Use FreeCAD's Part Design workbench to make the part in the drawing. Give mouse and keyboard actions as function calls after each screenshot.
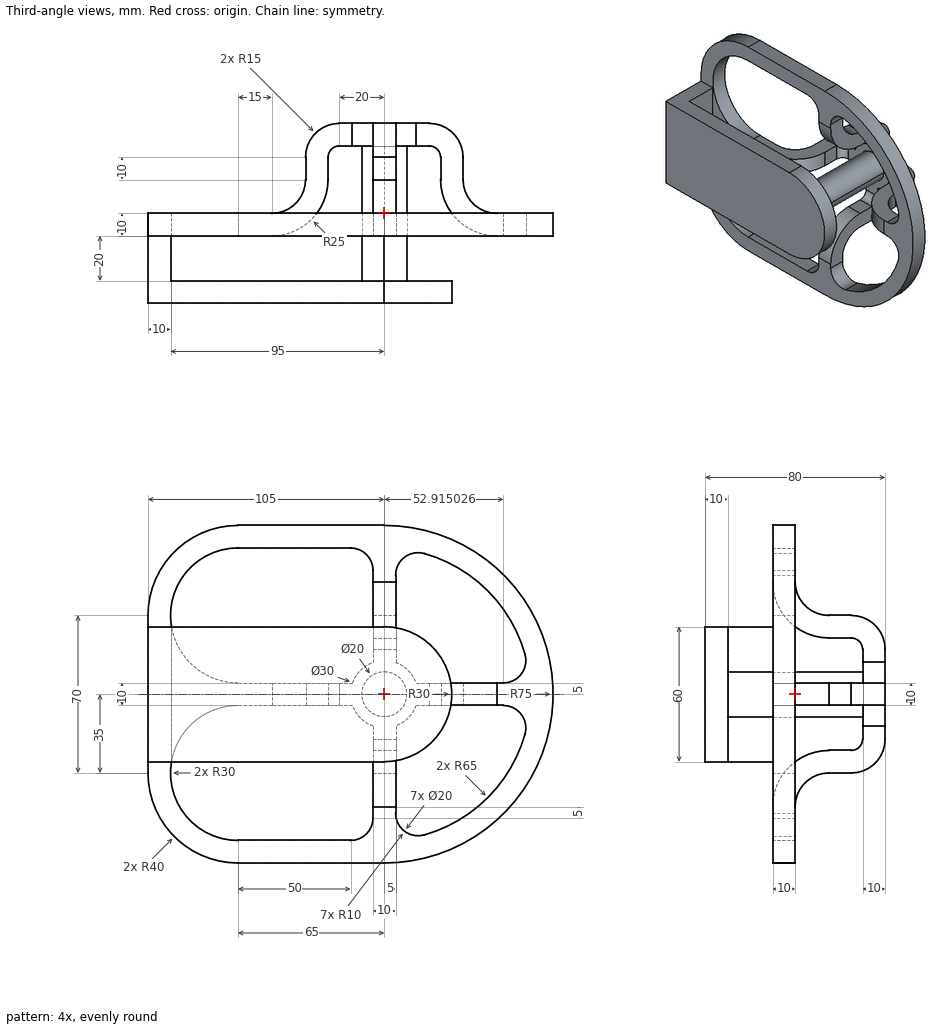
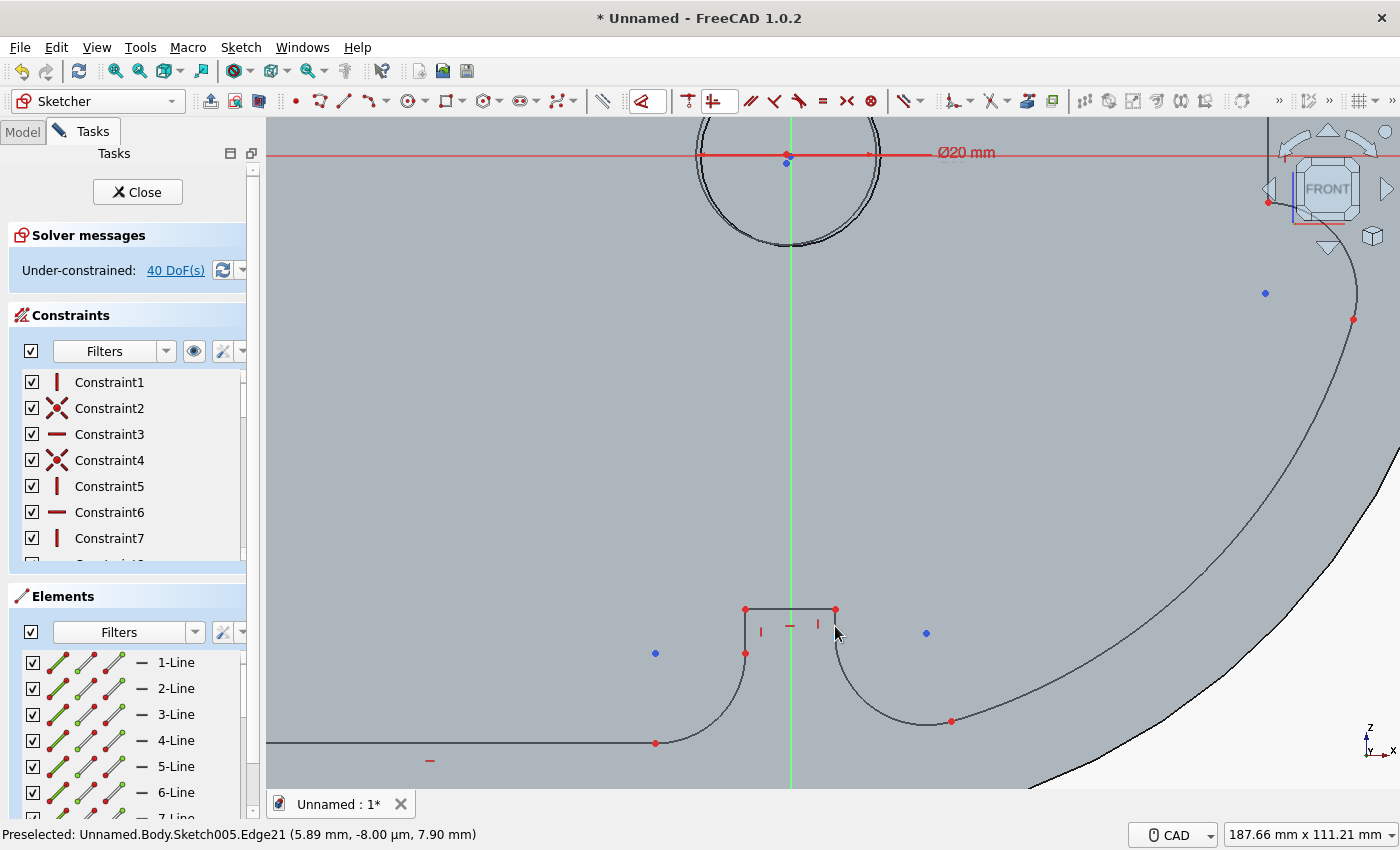
click(835, 623)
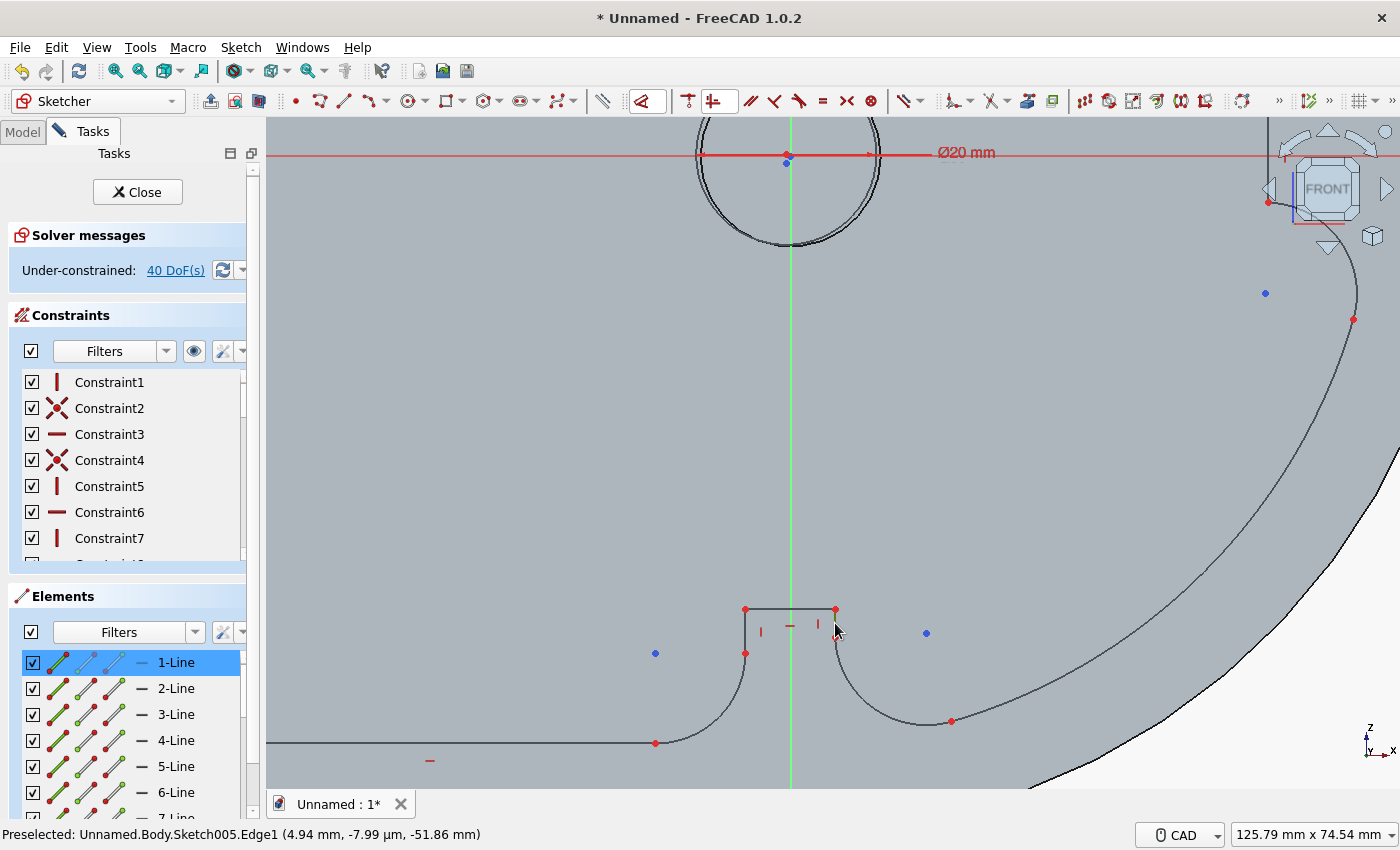
click(850, 684)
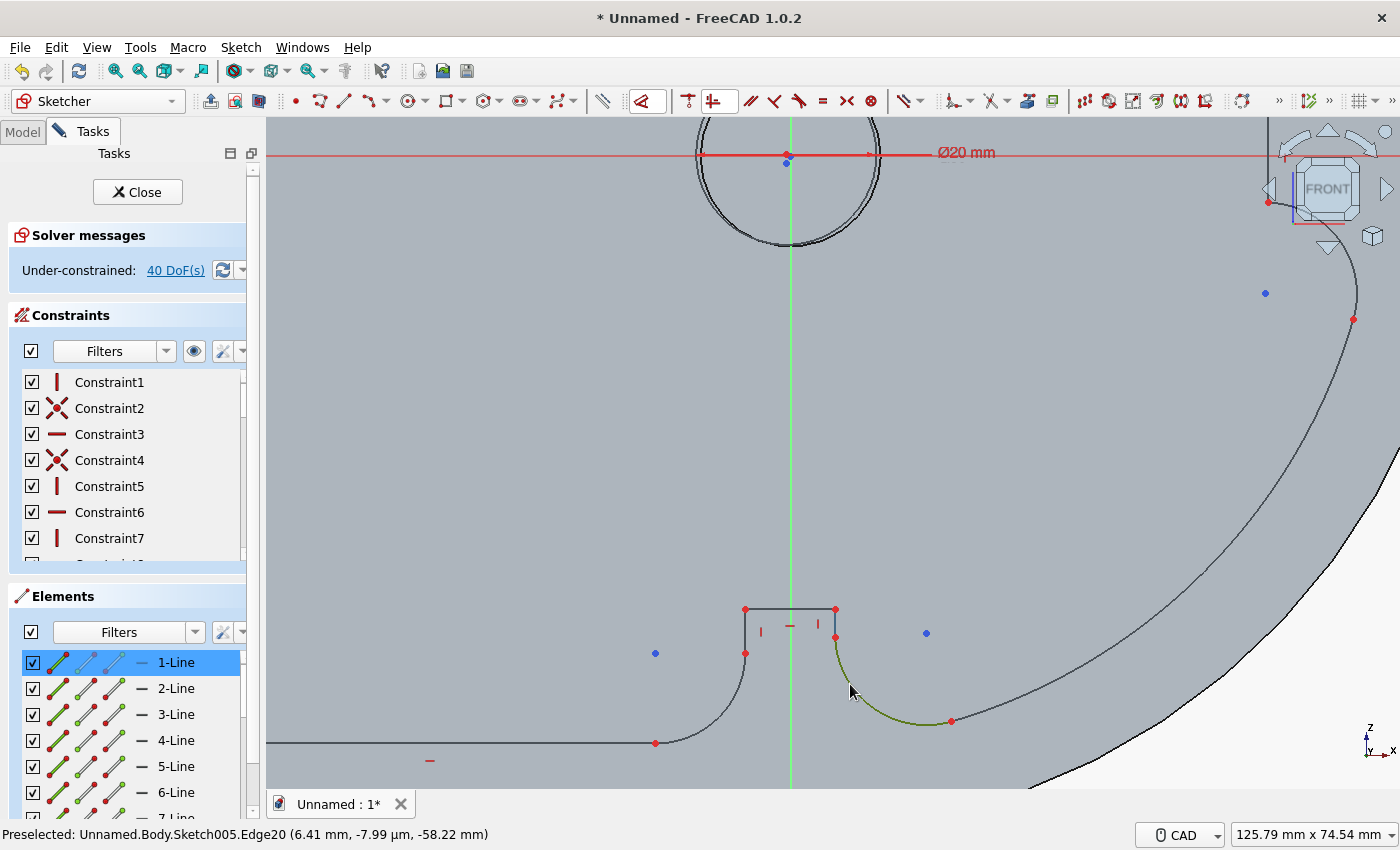
click(800, 102)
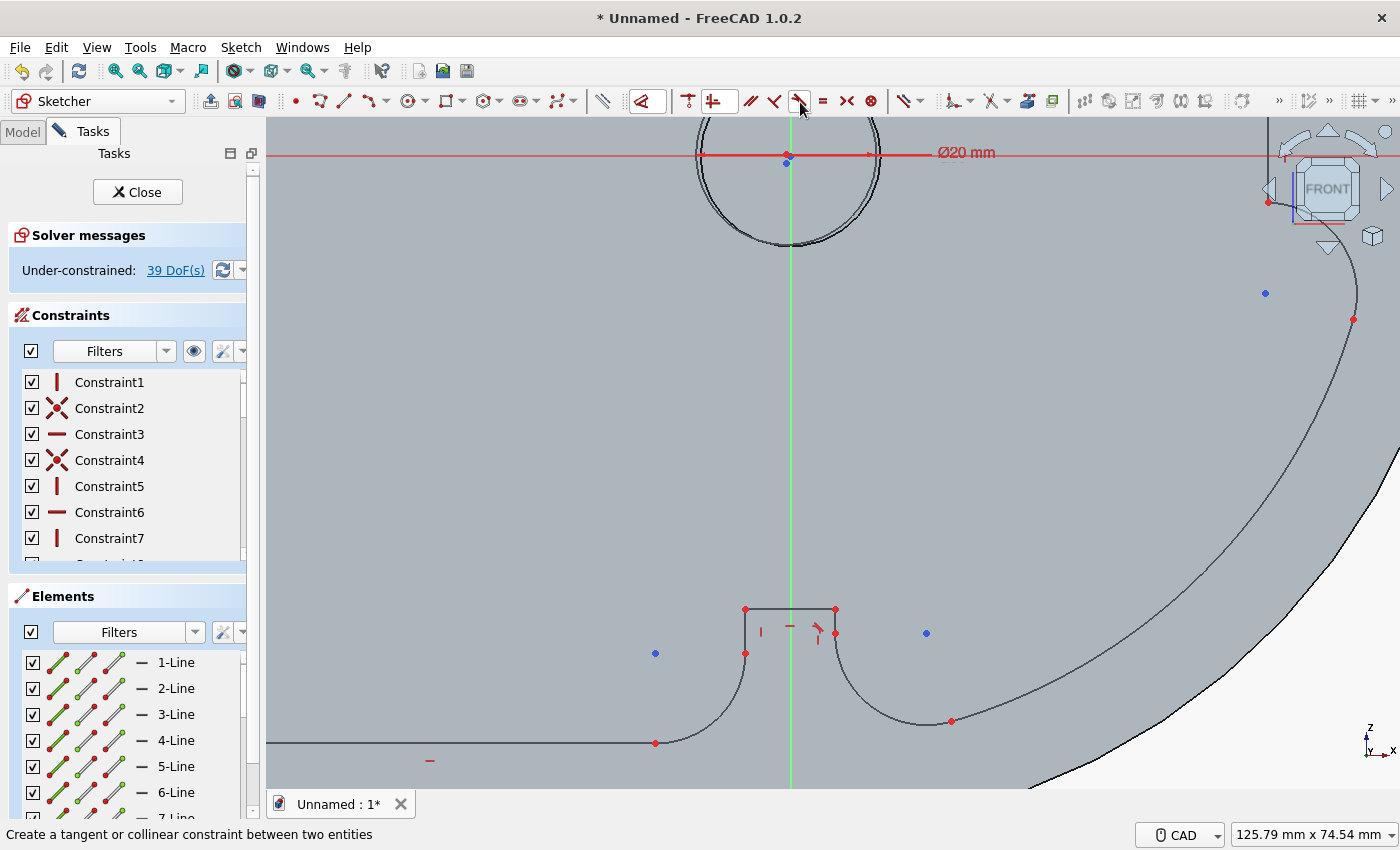
click(745, 623)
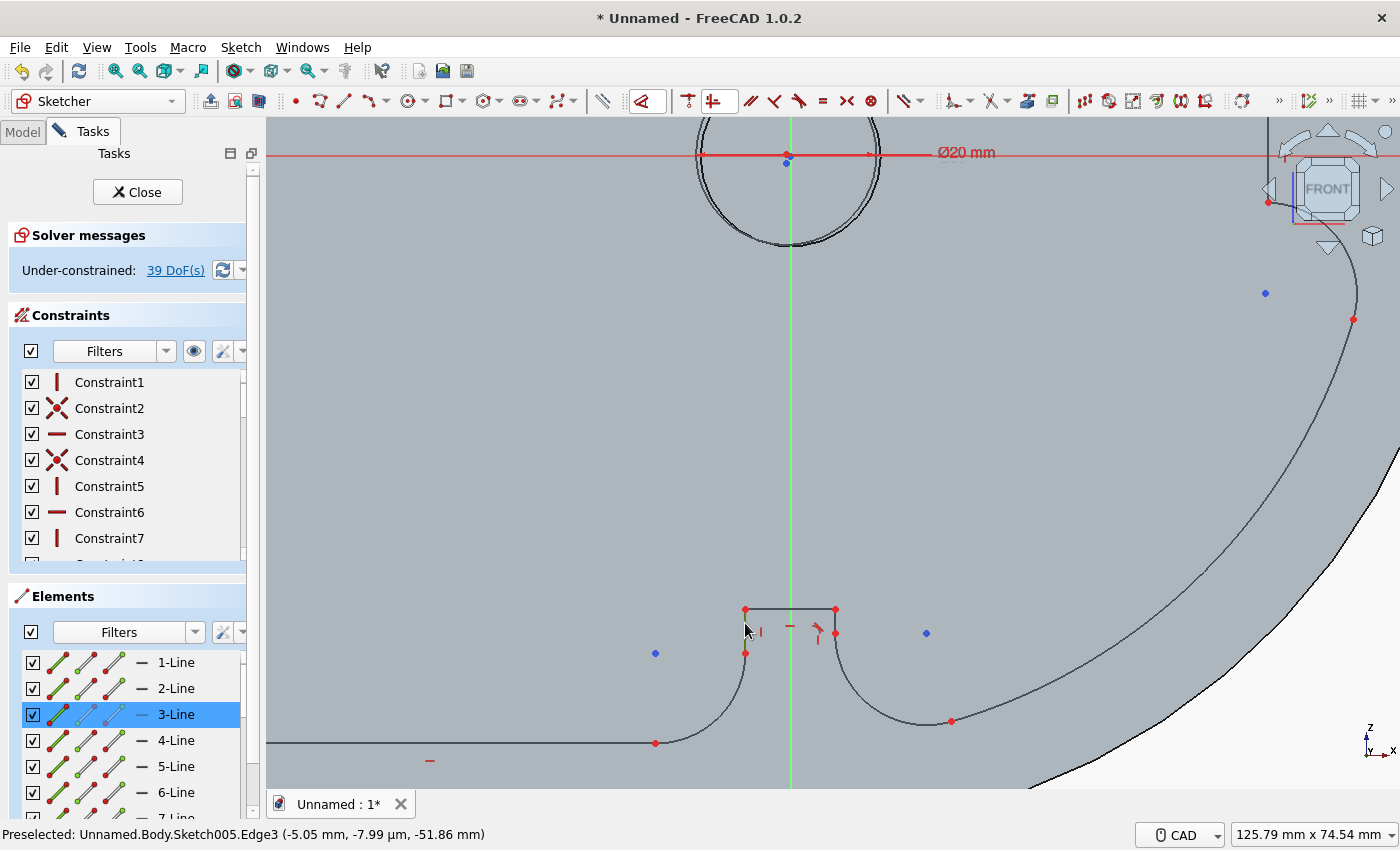
click(696, 734)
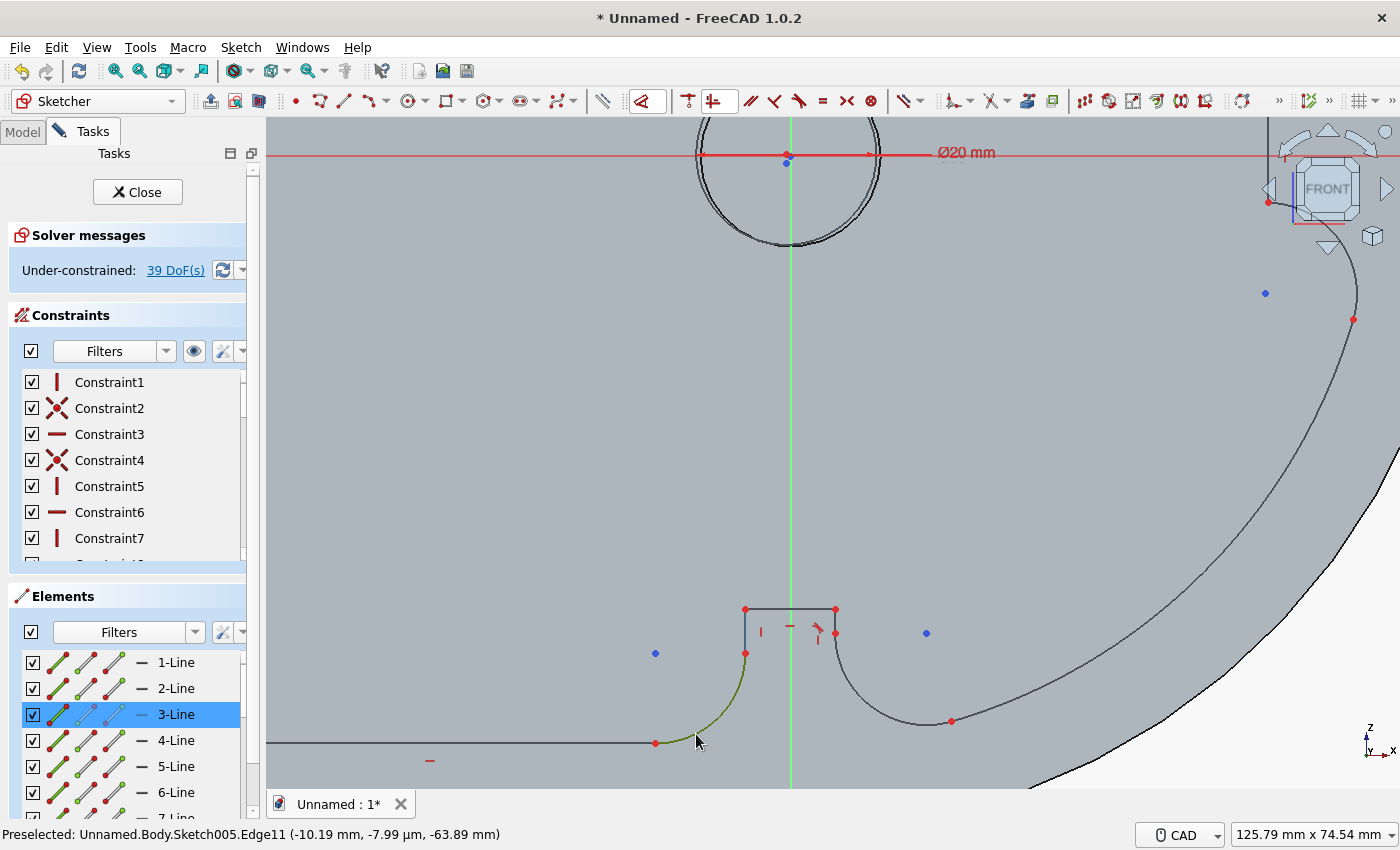
click(800, 102)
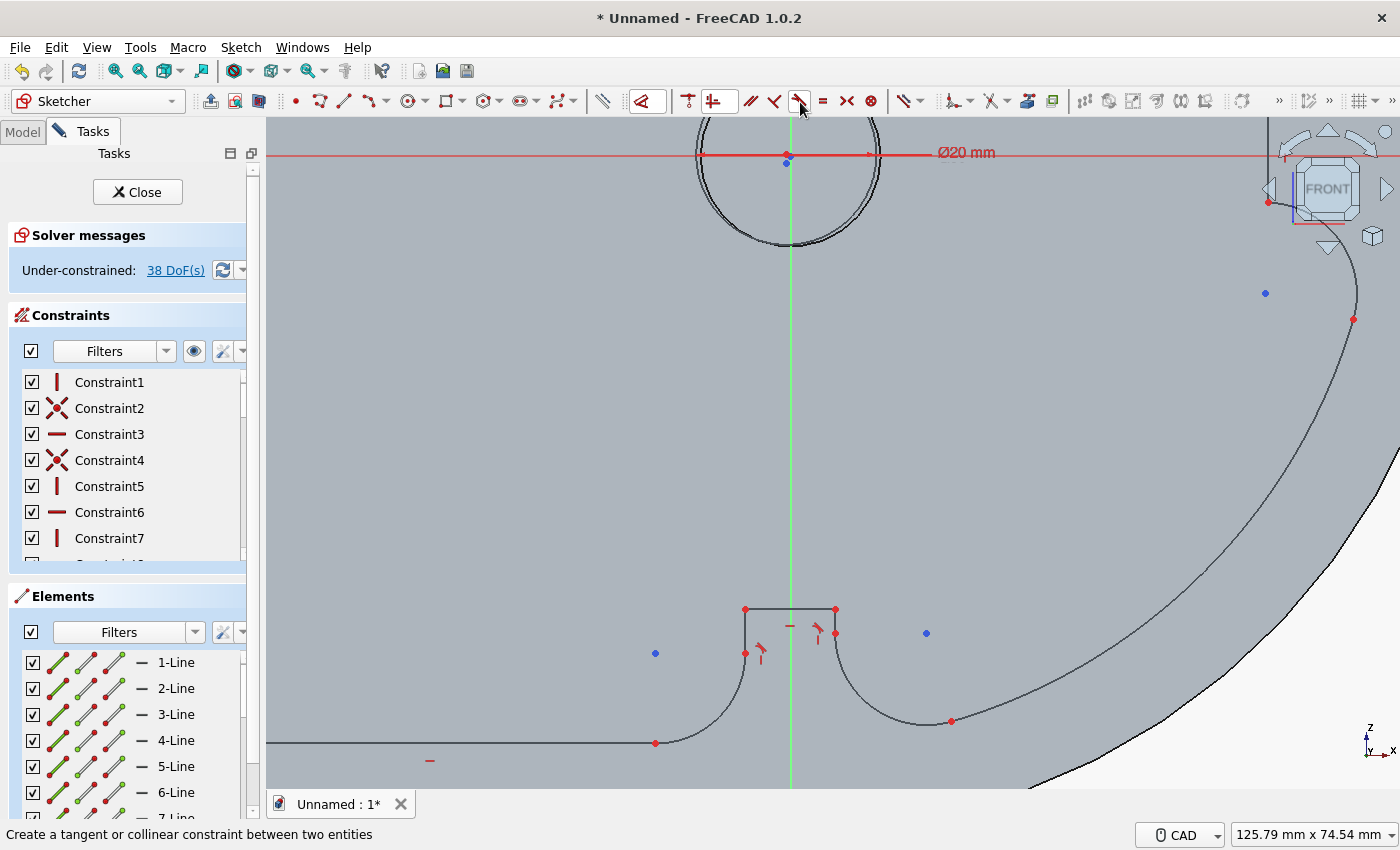
click(520, 743)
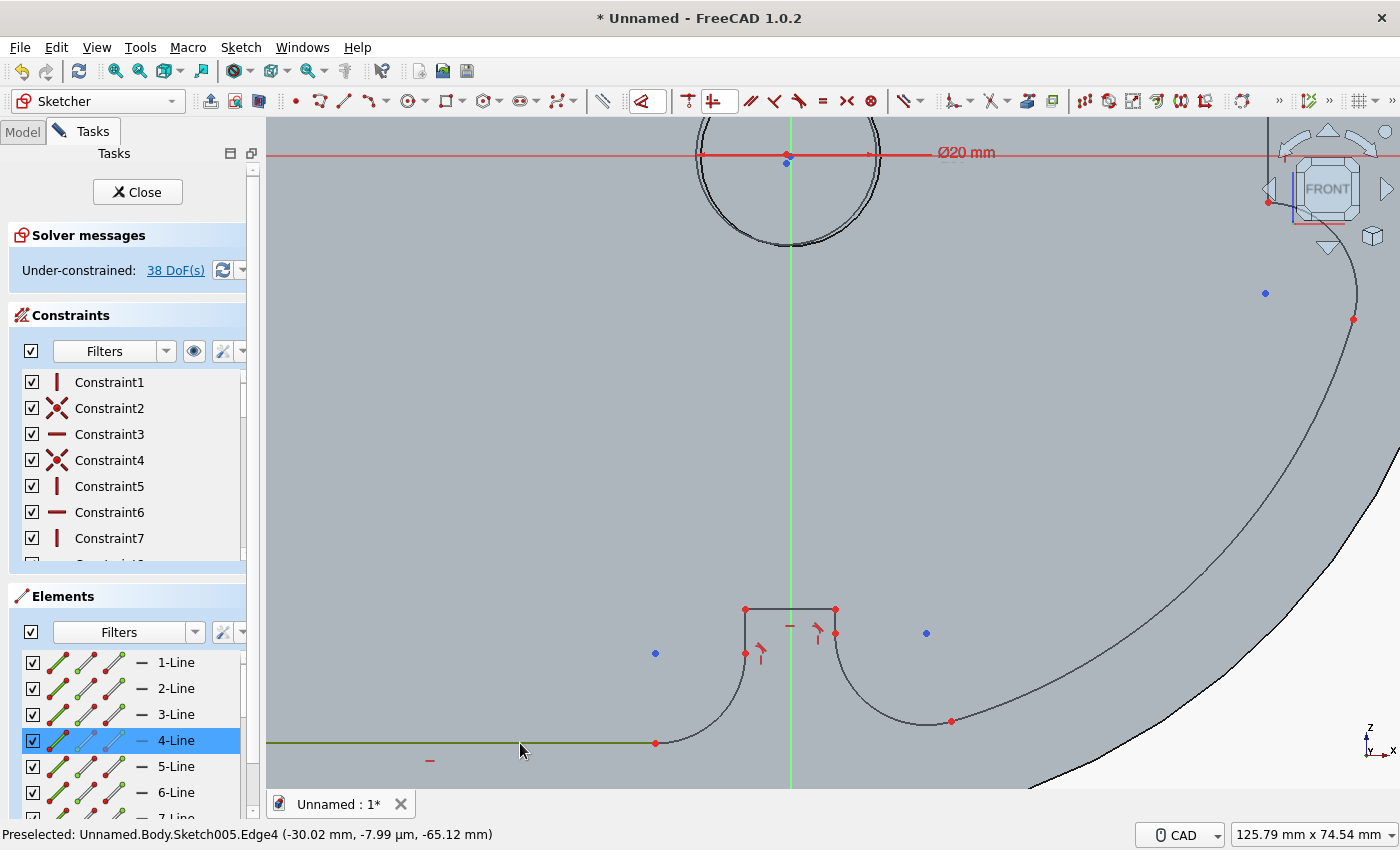
click(696, 734)